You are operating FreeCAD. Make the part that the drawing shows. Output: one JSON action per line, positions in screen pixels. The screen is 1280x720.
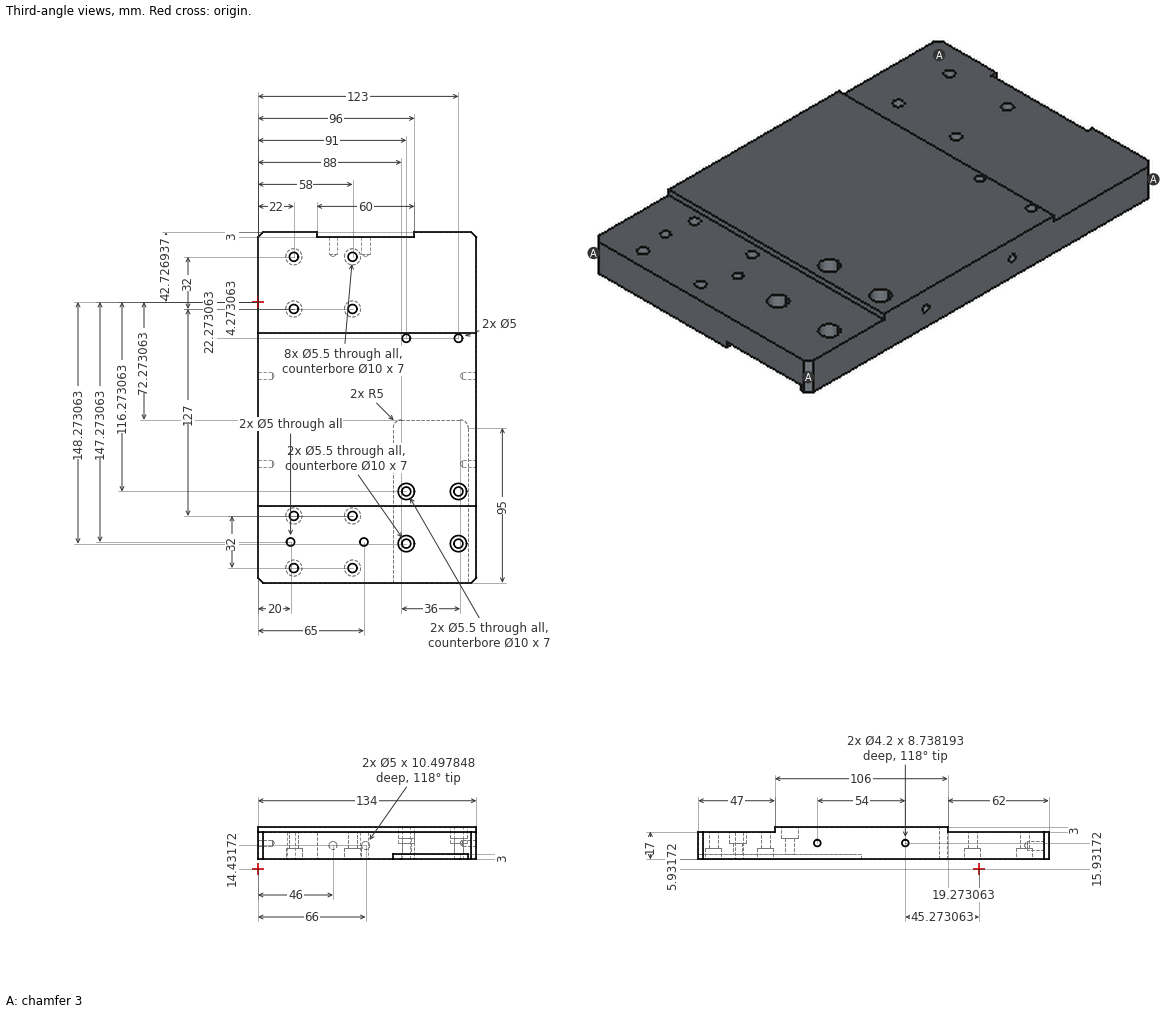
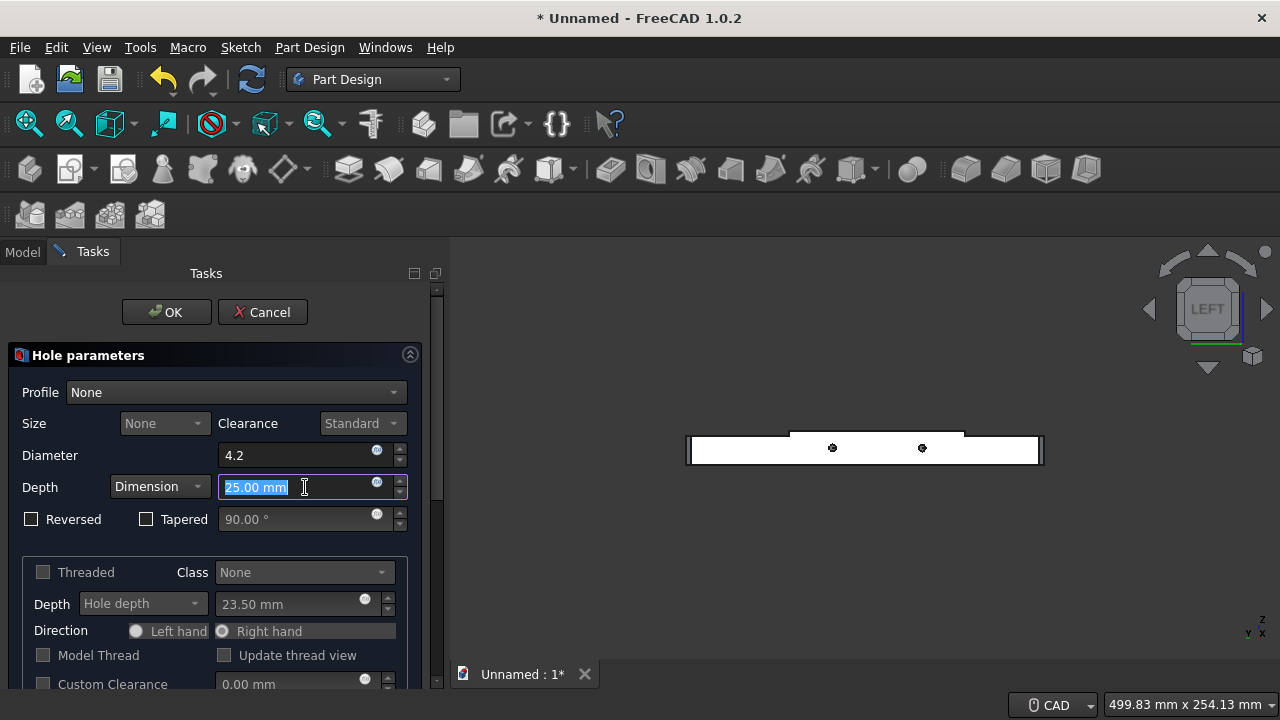
{"action": "type", "text": "8.738193"}
{"action": "key", "text": "Tab"}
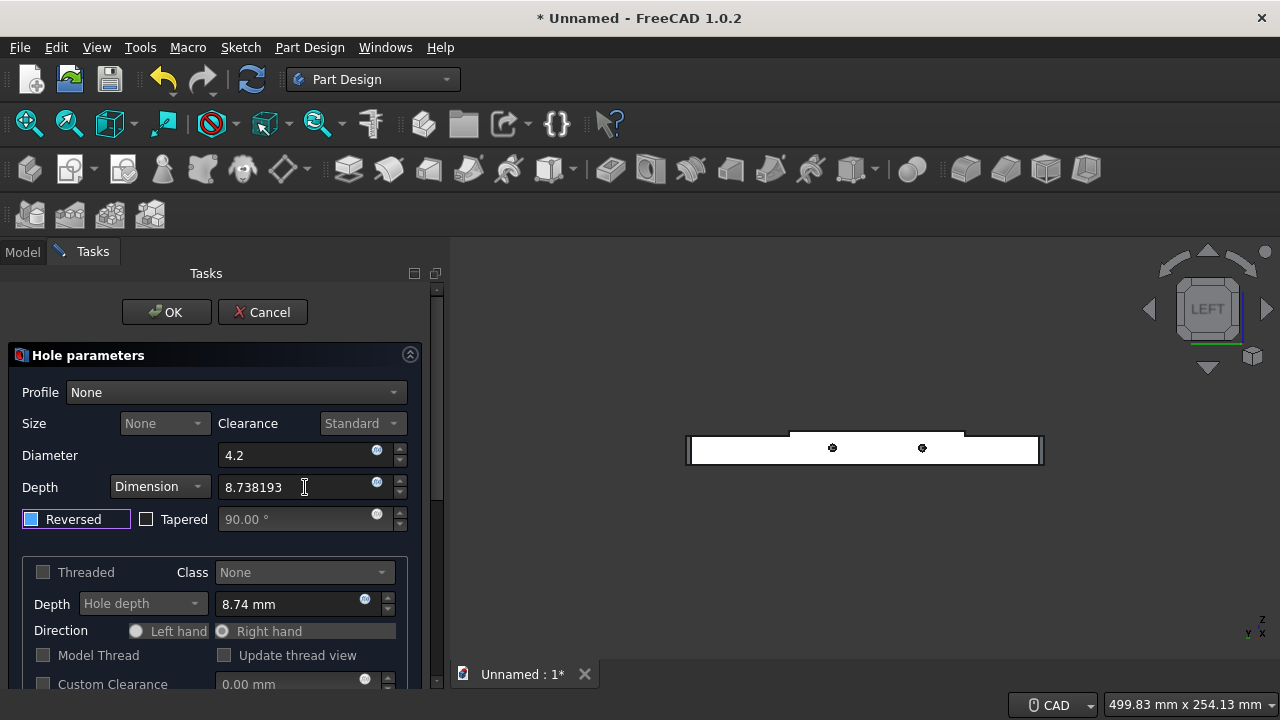
{"action": "left_click", "coordinate": [167, 312]}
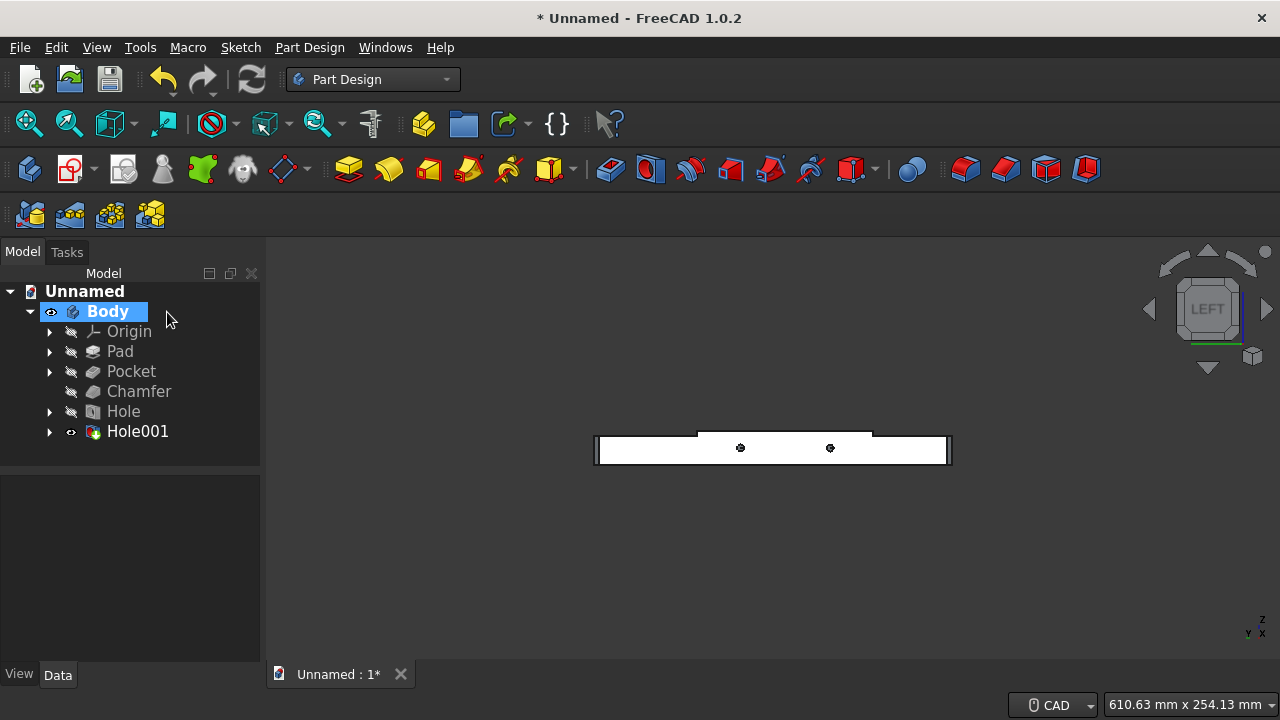
{"action": "left_click", "coordinate": [30, 124]}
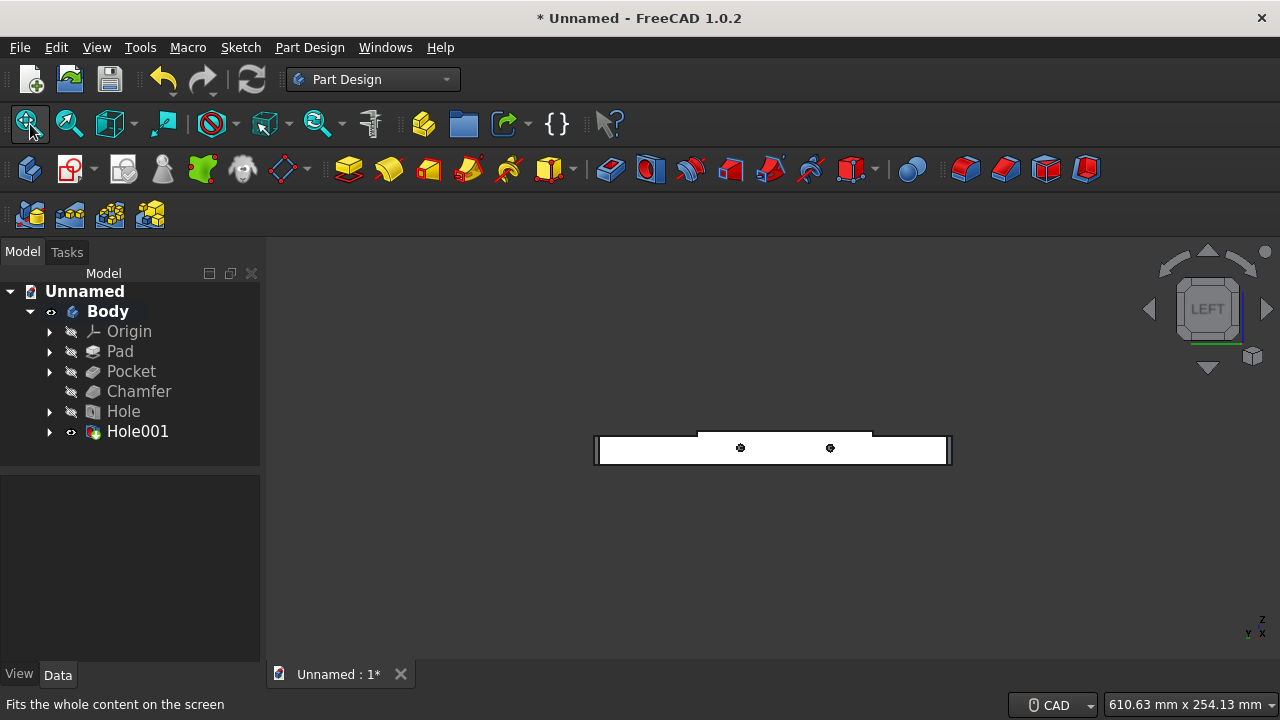
{"action": "key", "text": "4"}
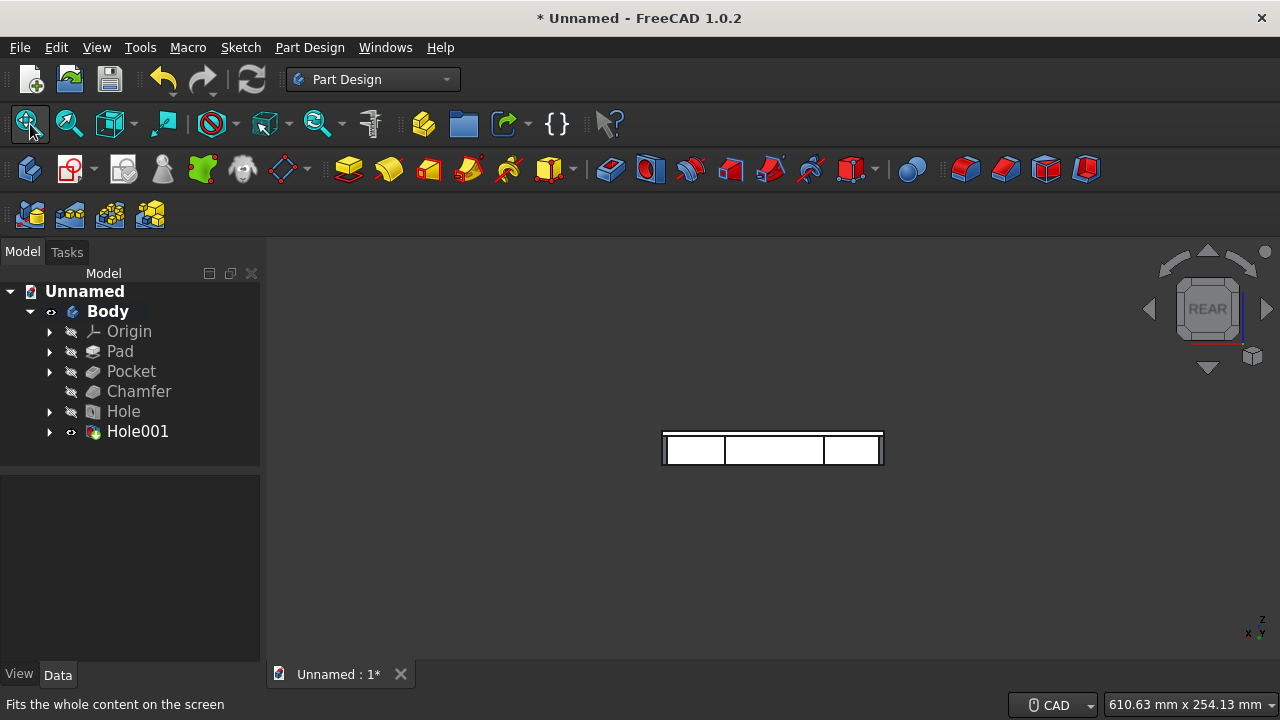
{"action": "left_click", "coordinate": [30, 124]}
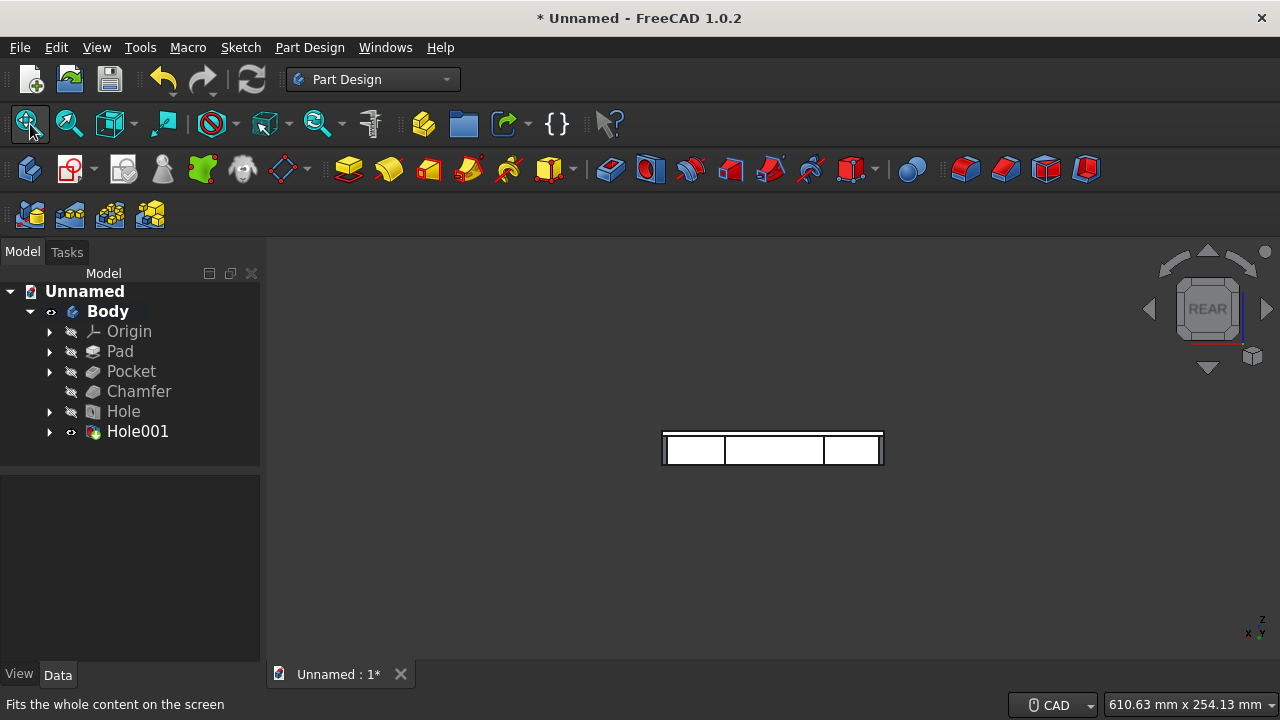
{"action": "left_click", "coordinate": [803, 449]}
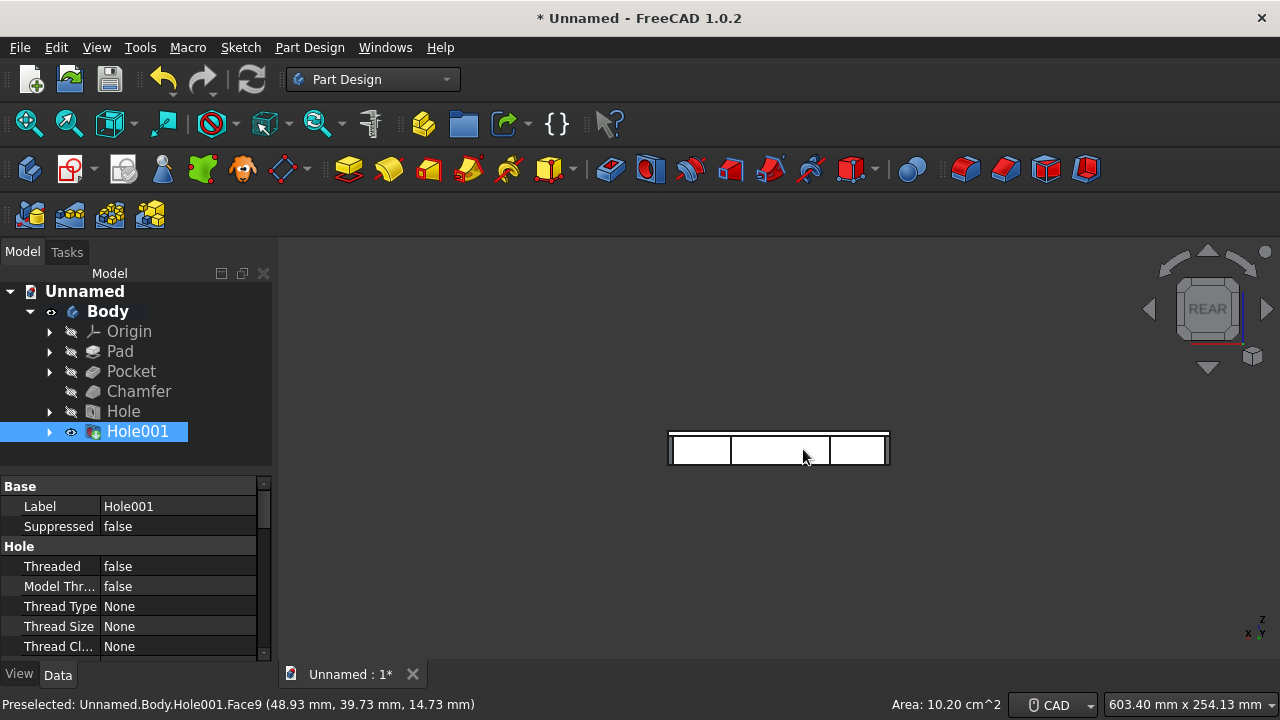
{"action": "left_click", "coordinate": [70, 170]}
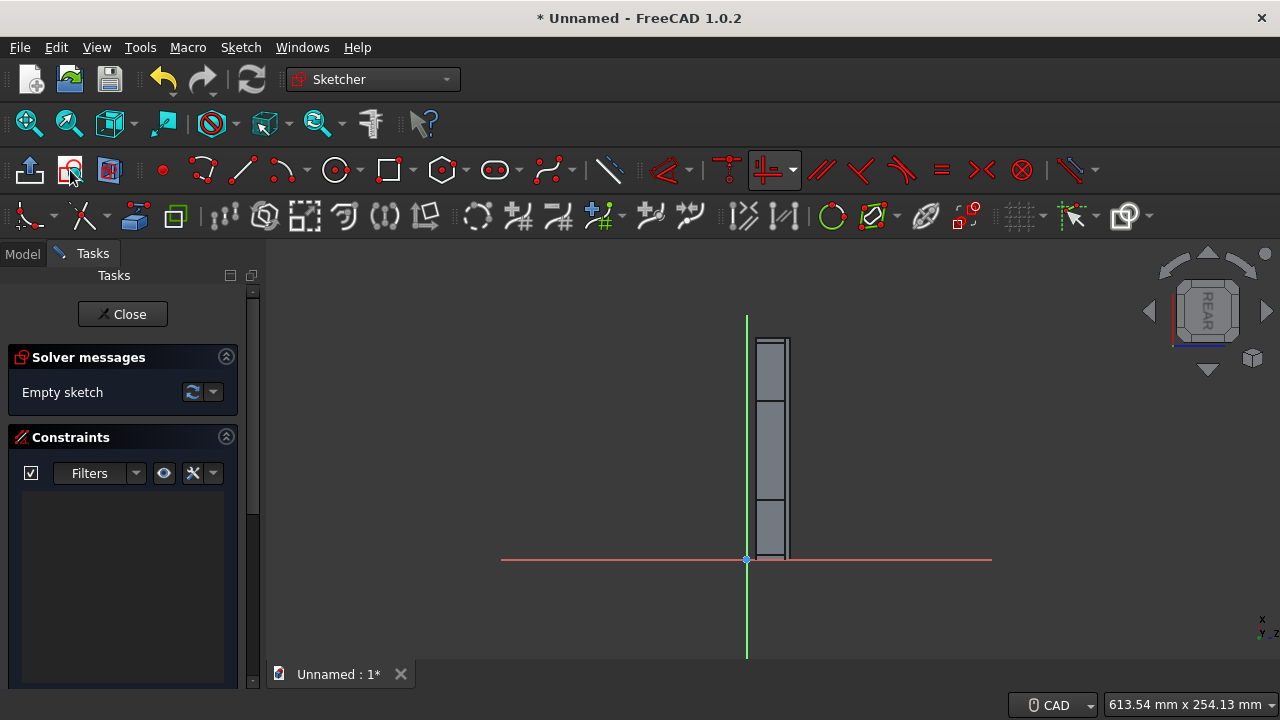
{"action": "left_click", "coordinate": [110, 170]}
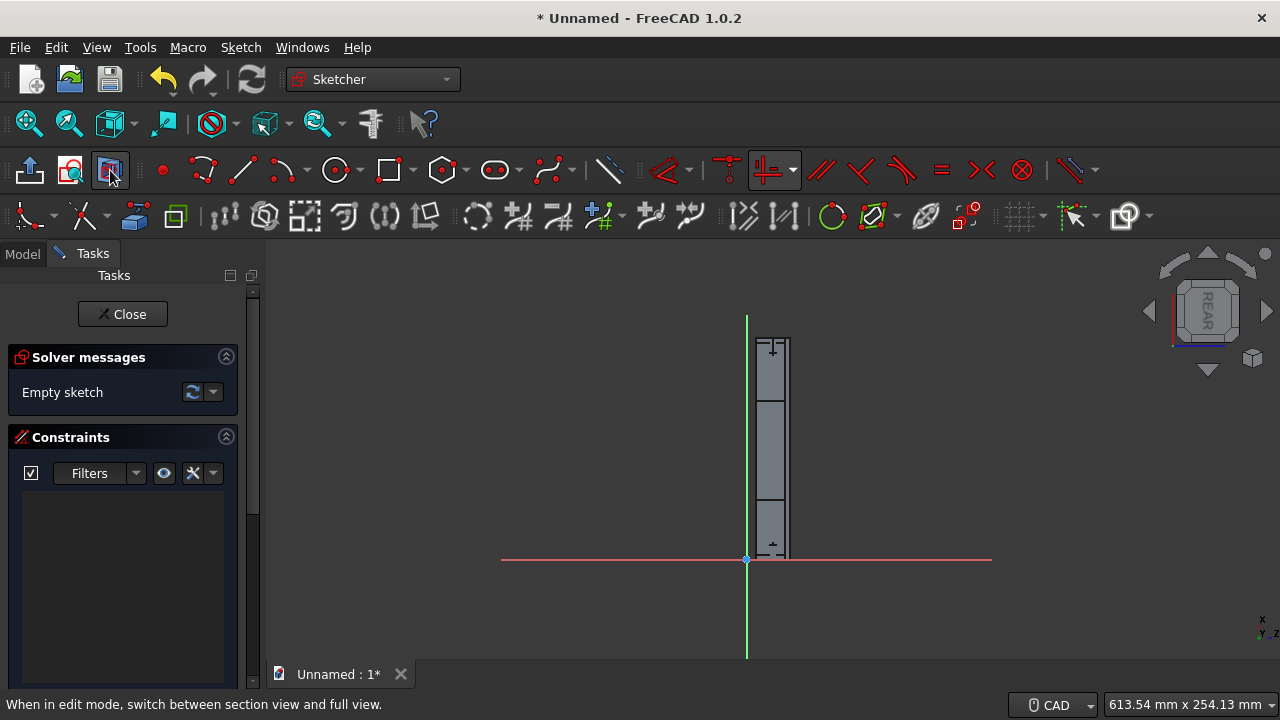
{"action": "scroll", "coordinate": [784, 471], "scroll_direction": "up", "scroll_amount": 9}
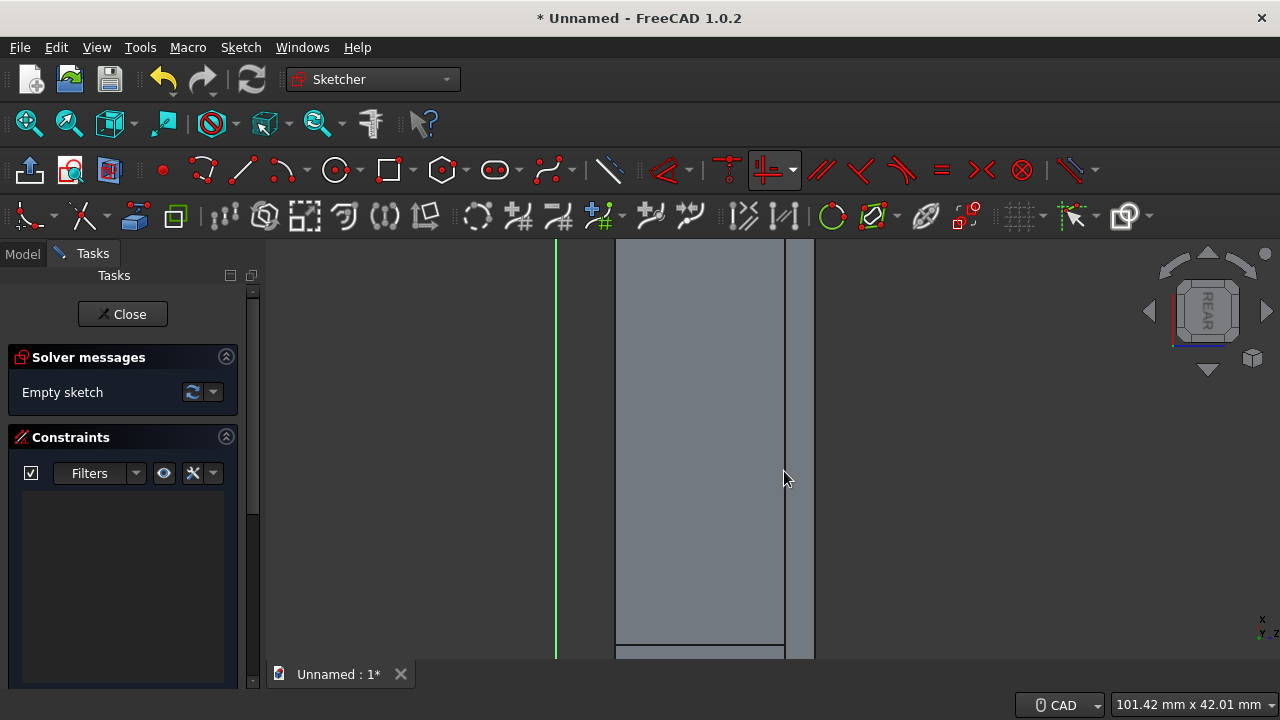
{"action": "left_click", "coordinate": [336, 170]}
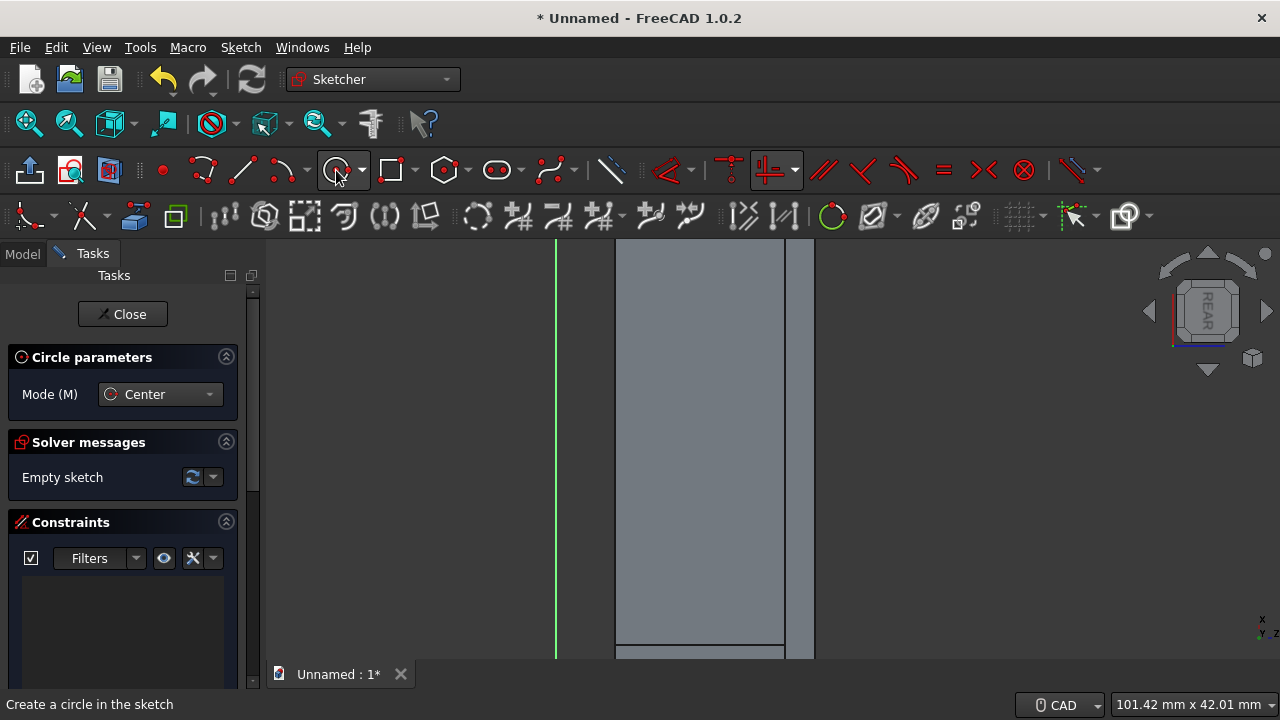
{"action": "left_click", "coordinate": [700, 345]}
{"action": "mouse_move", "coordinate": [718, 327]}